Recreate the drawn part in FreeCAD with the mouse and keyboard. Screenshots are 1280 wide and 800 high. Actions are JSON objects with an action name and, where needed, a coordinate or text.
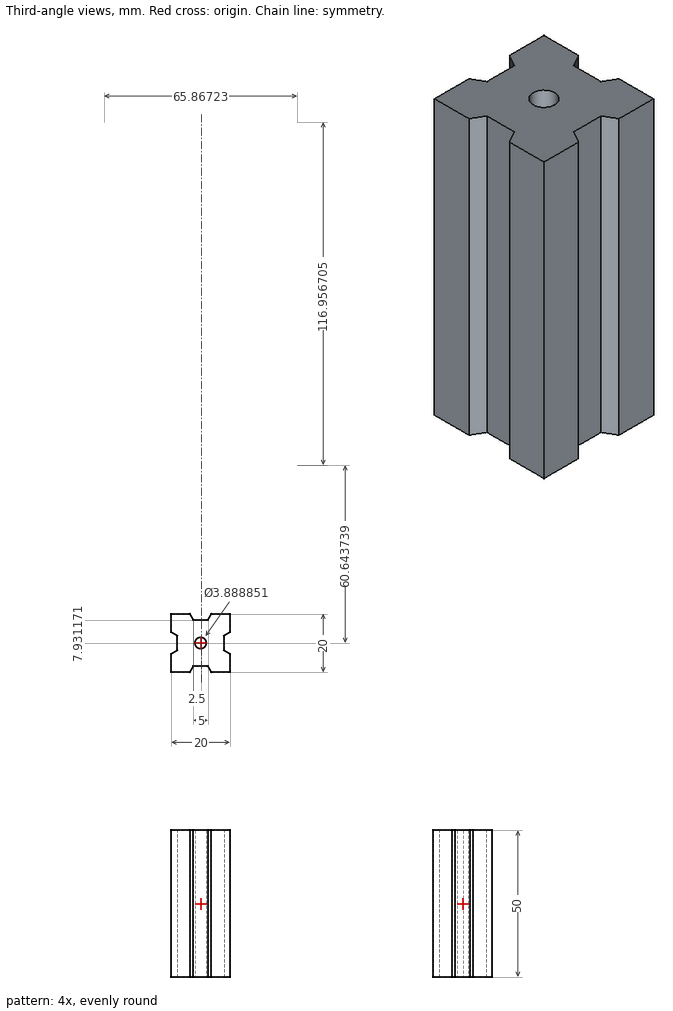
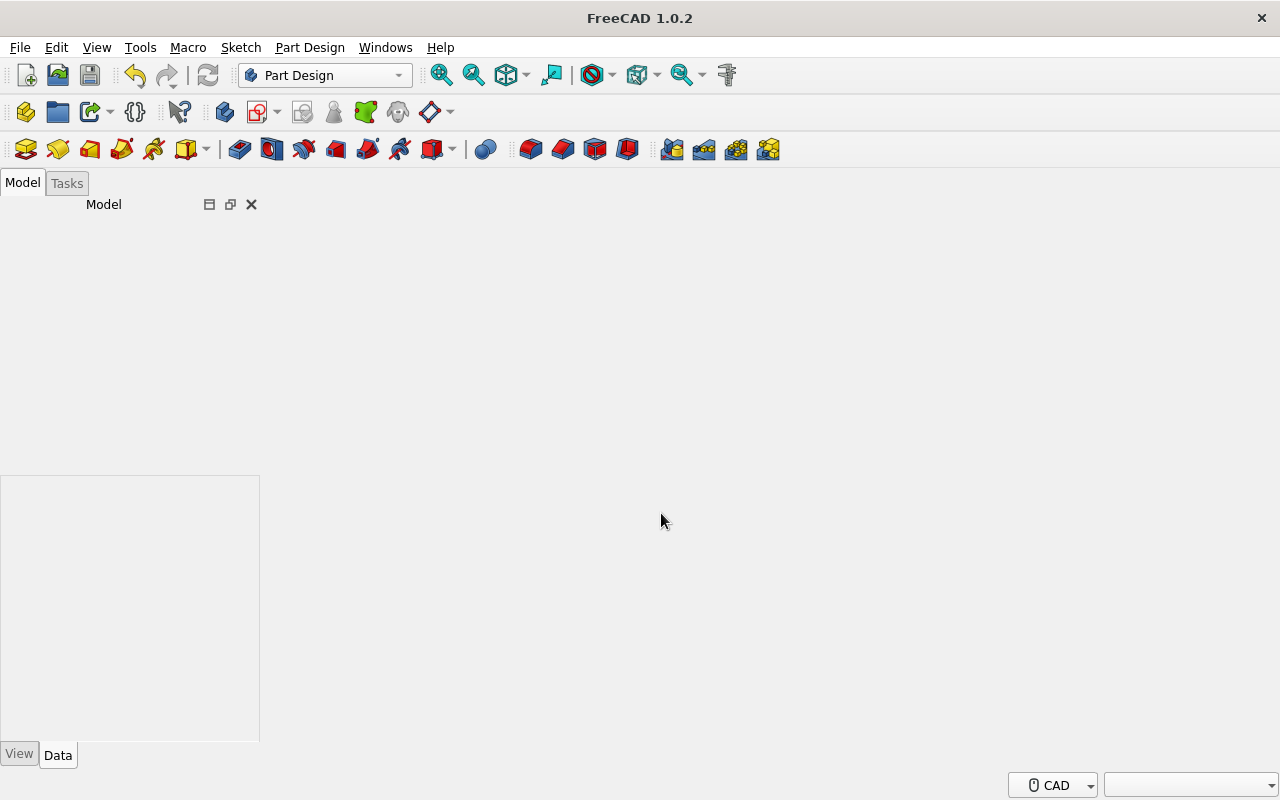
{"action": "key", "text": "ctrl+n"}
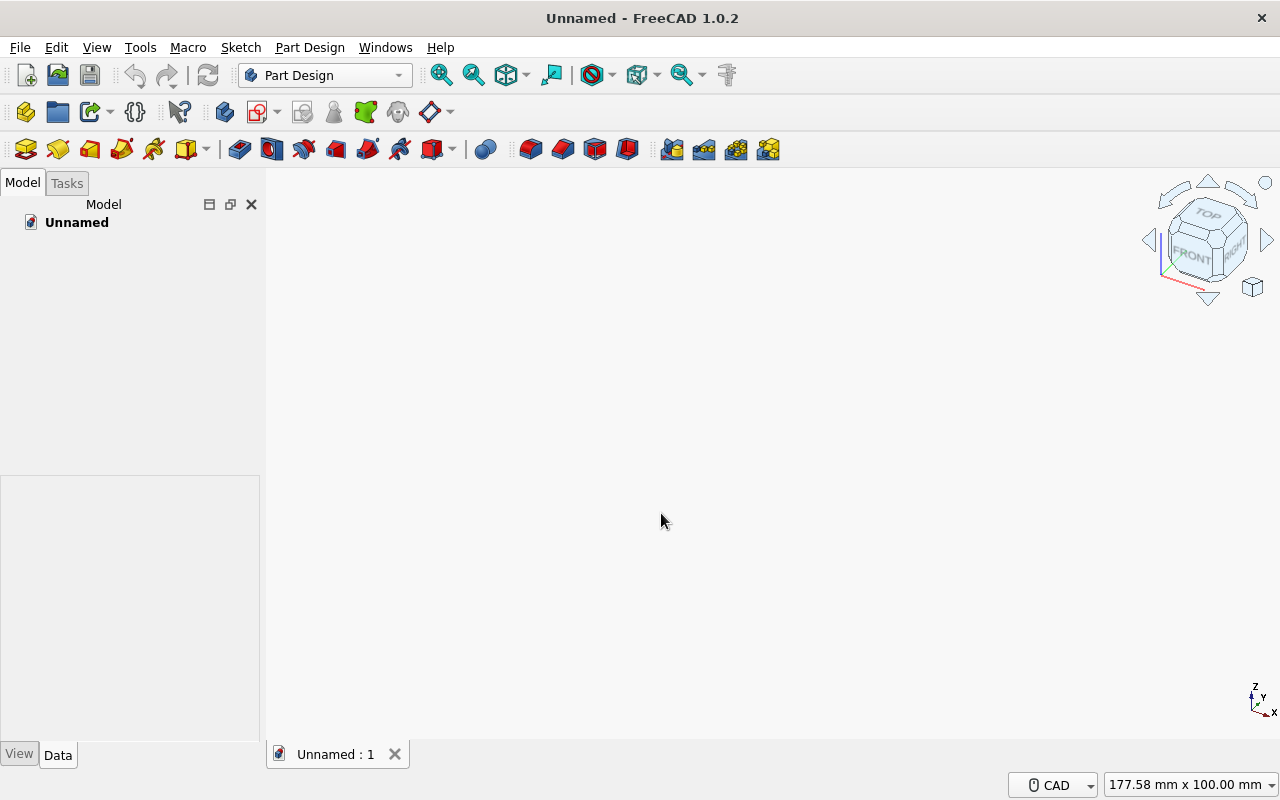
{"action": "left_click", "coordinate": [258, 112]}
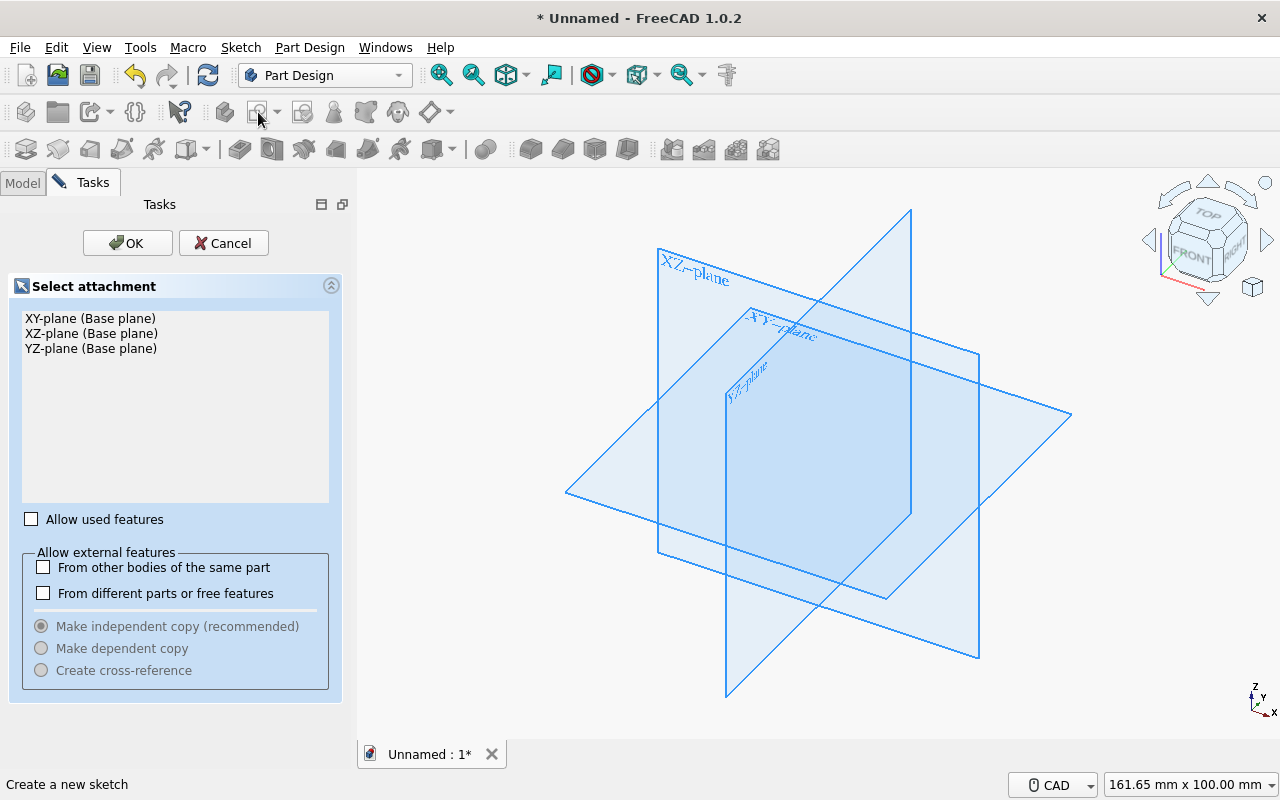
{"action": "left_click", "coordinate": [82, 318]}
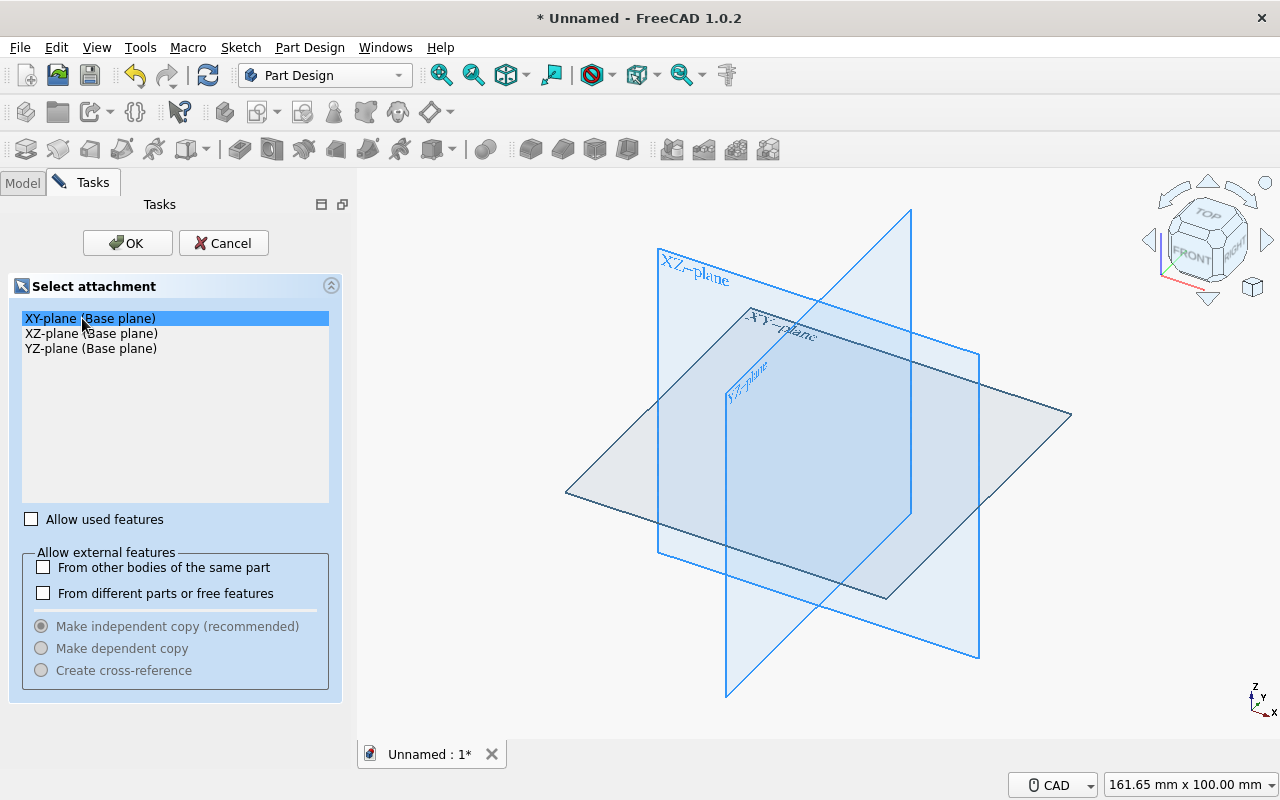
{"action": "left_click", "coordinate": [128, 243]}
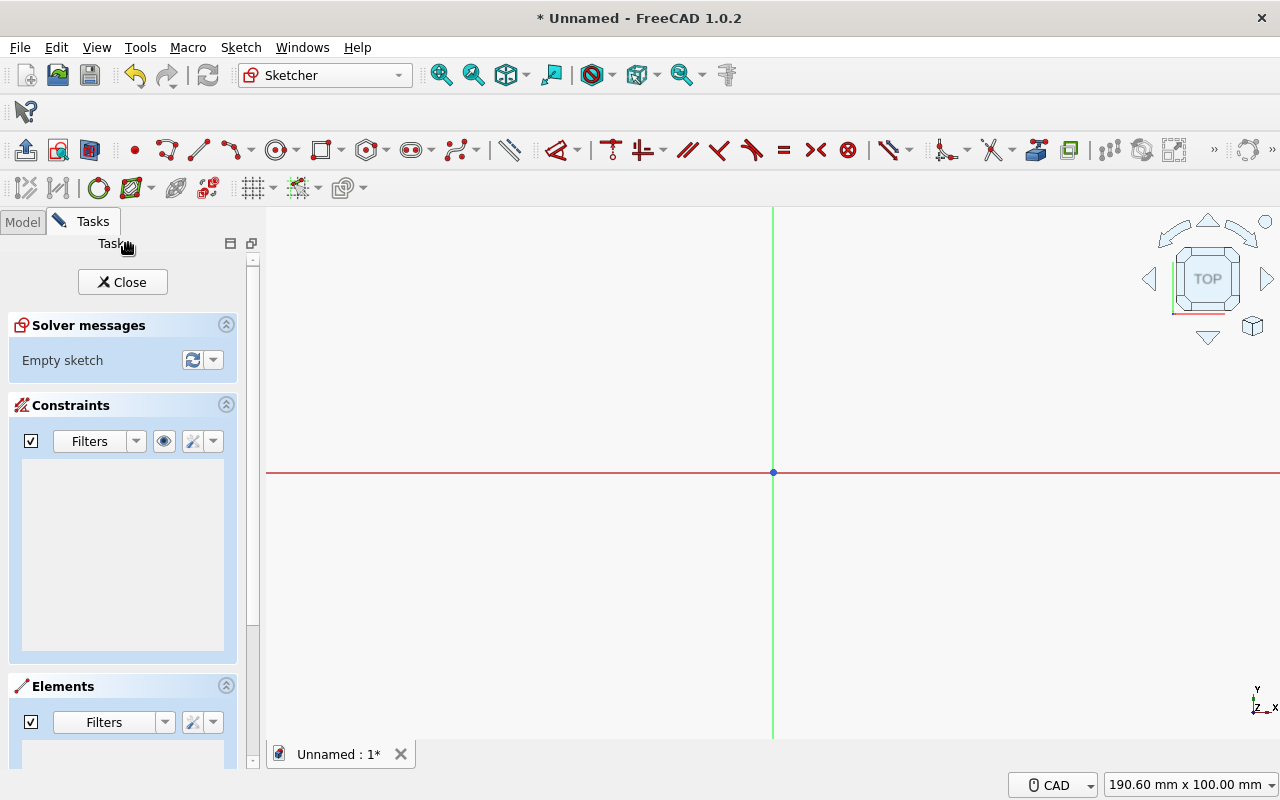
{"action": "scroll", "coordinate": [803, 473], "scroll_direction": "up", "scroll_amount": 6}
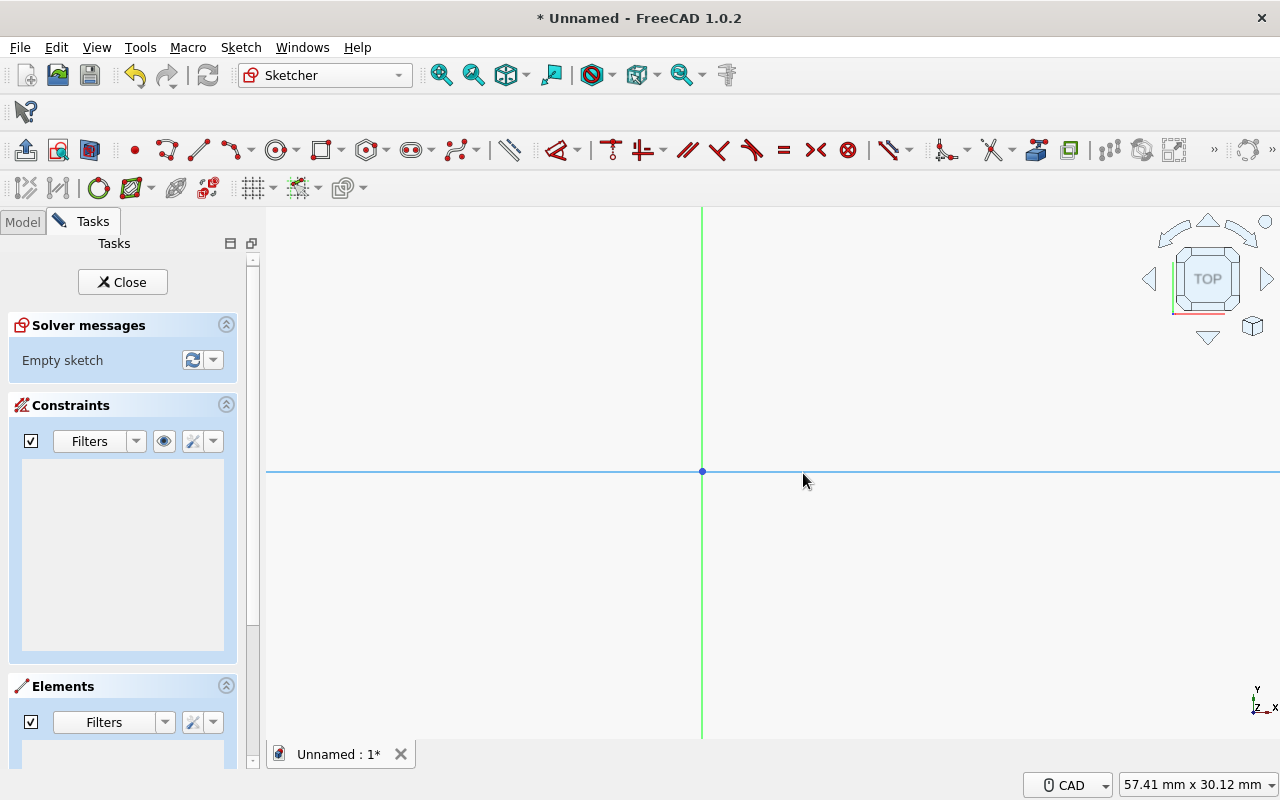
{"action": "key", "text": "g v"}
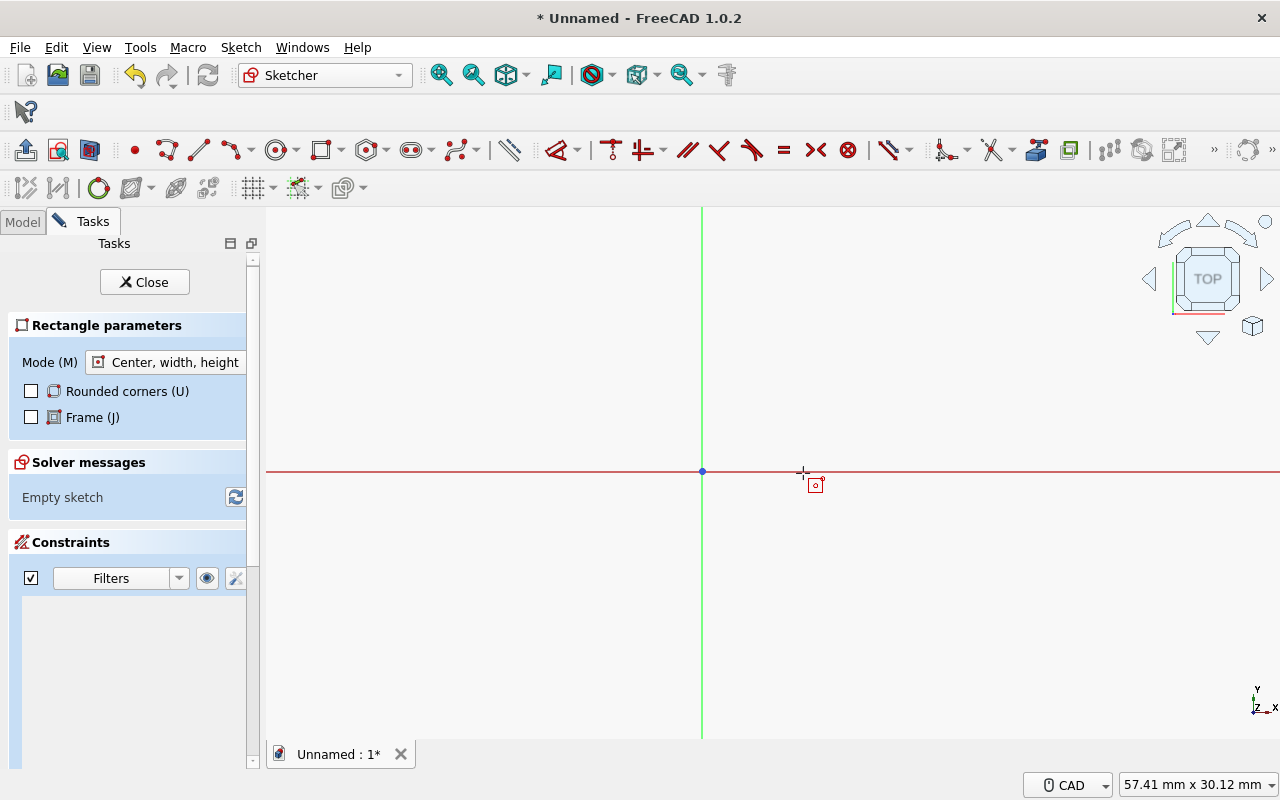
{"action": "left_click", "coordinate": [702, 472]}
{"action": "left_click", "coordinate": [879, 295]}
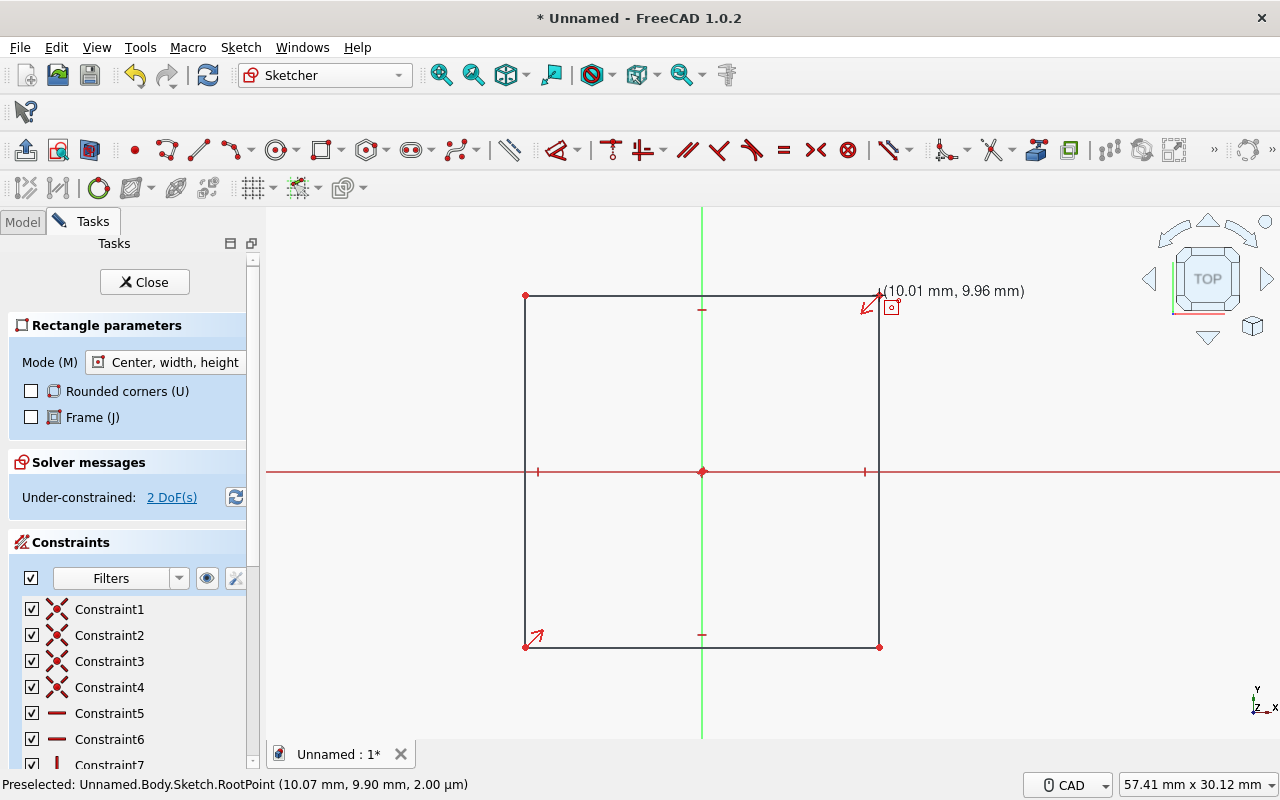
{"action": "left_click", "coordinate": [276, 150]}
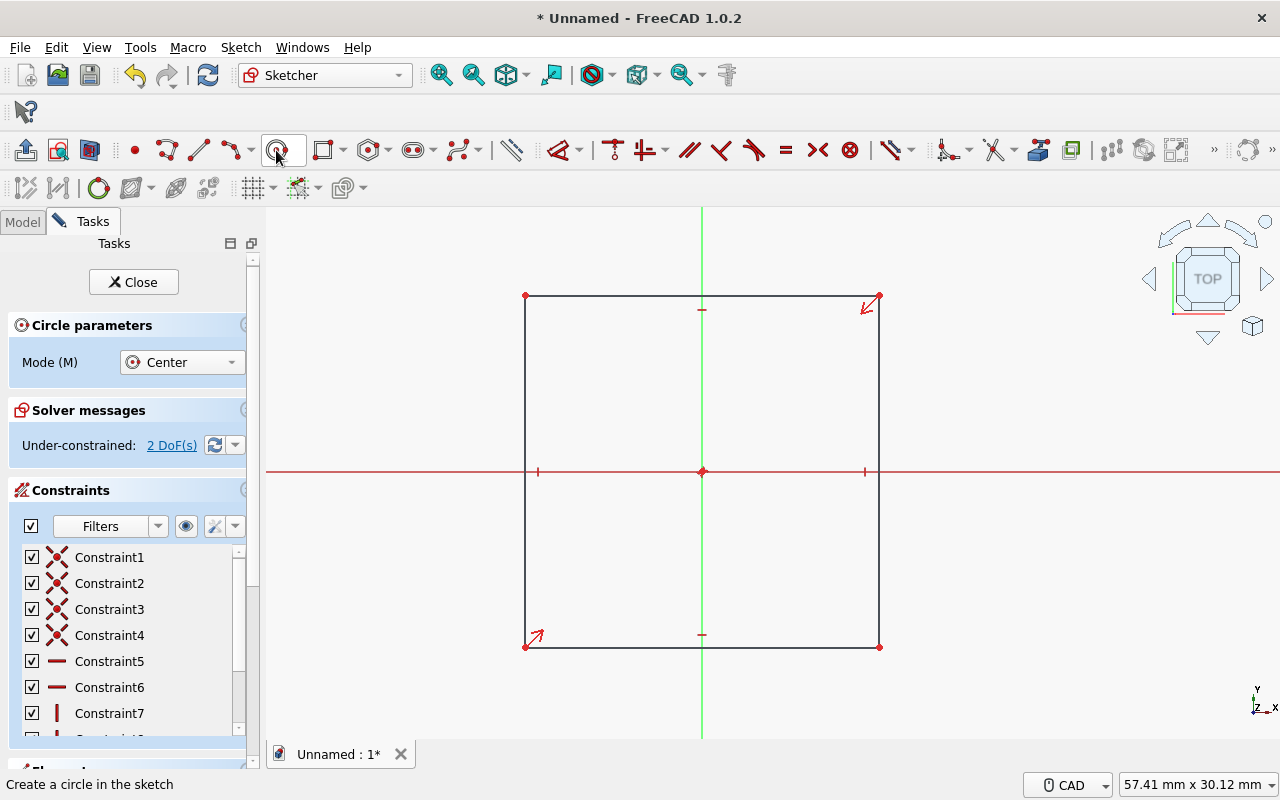
{"action": "left_click", "coordinate": [702, 472]}
{"action": "left_click", "coordinate": [726, 448]}
{"action": "key", "text": "Escape"}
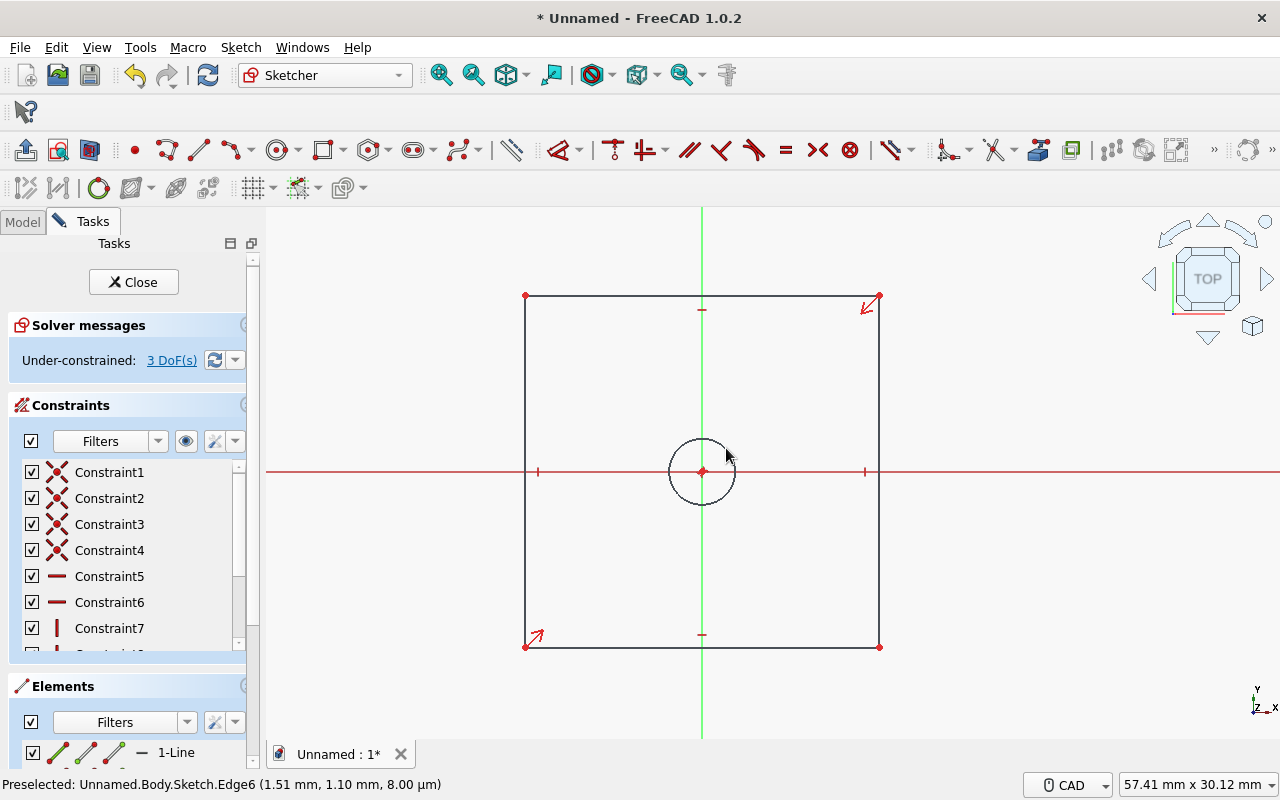
{"action": "left_click", "coordinate": [558, 150]}